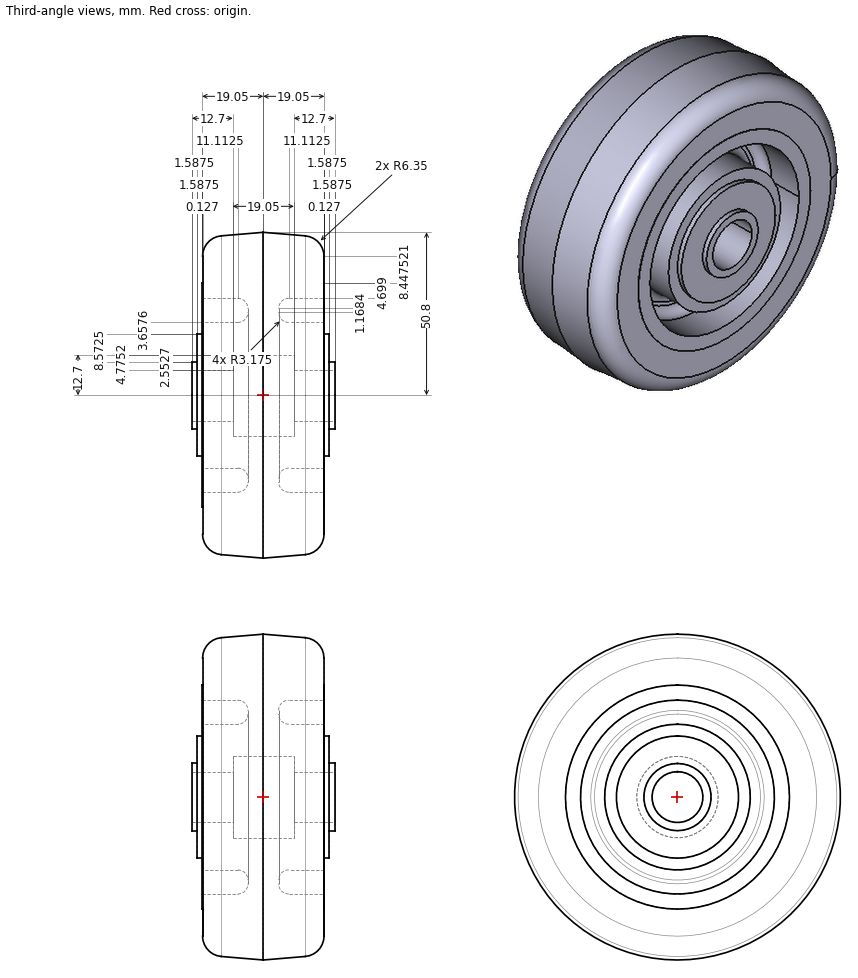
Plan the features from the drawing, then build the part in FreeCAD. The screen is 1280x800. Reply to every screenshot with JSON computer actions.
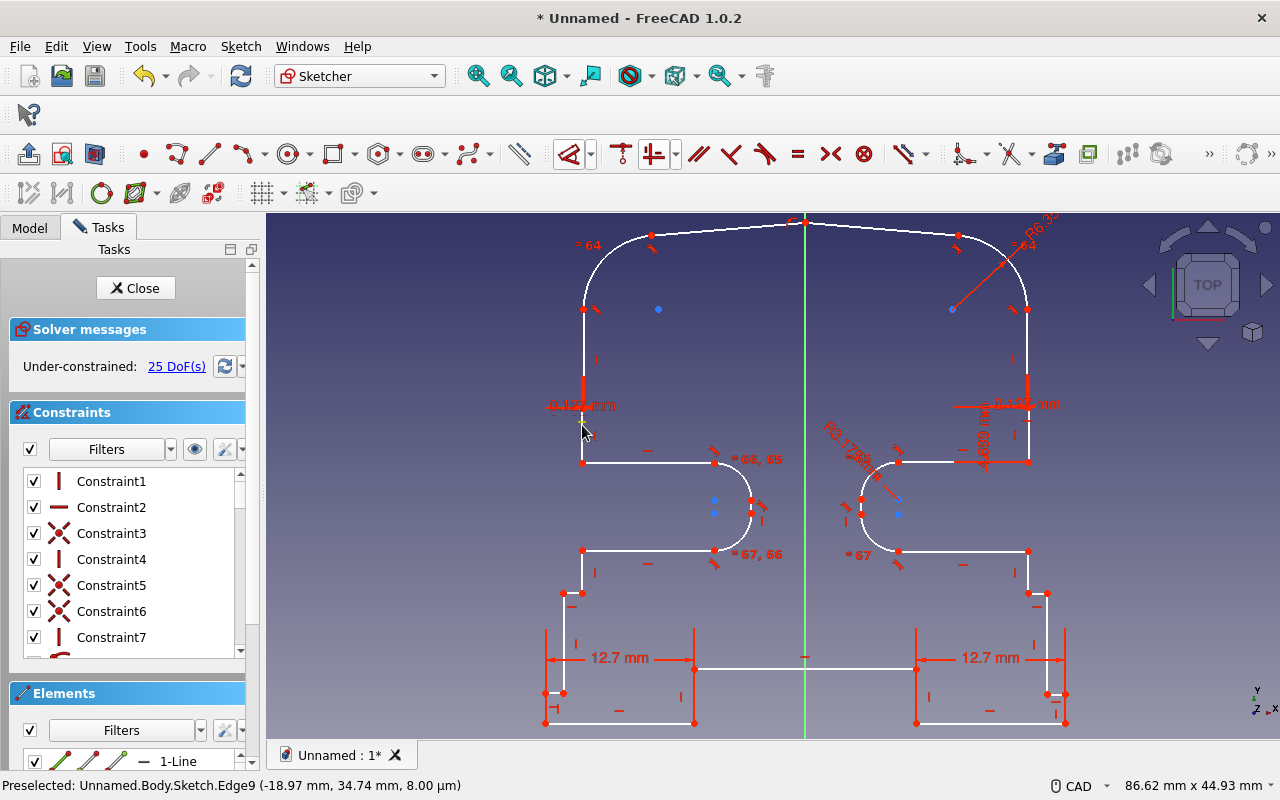
{"action": "left_click", "coordinate": [582, 447]}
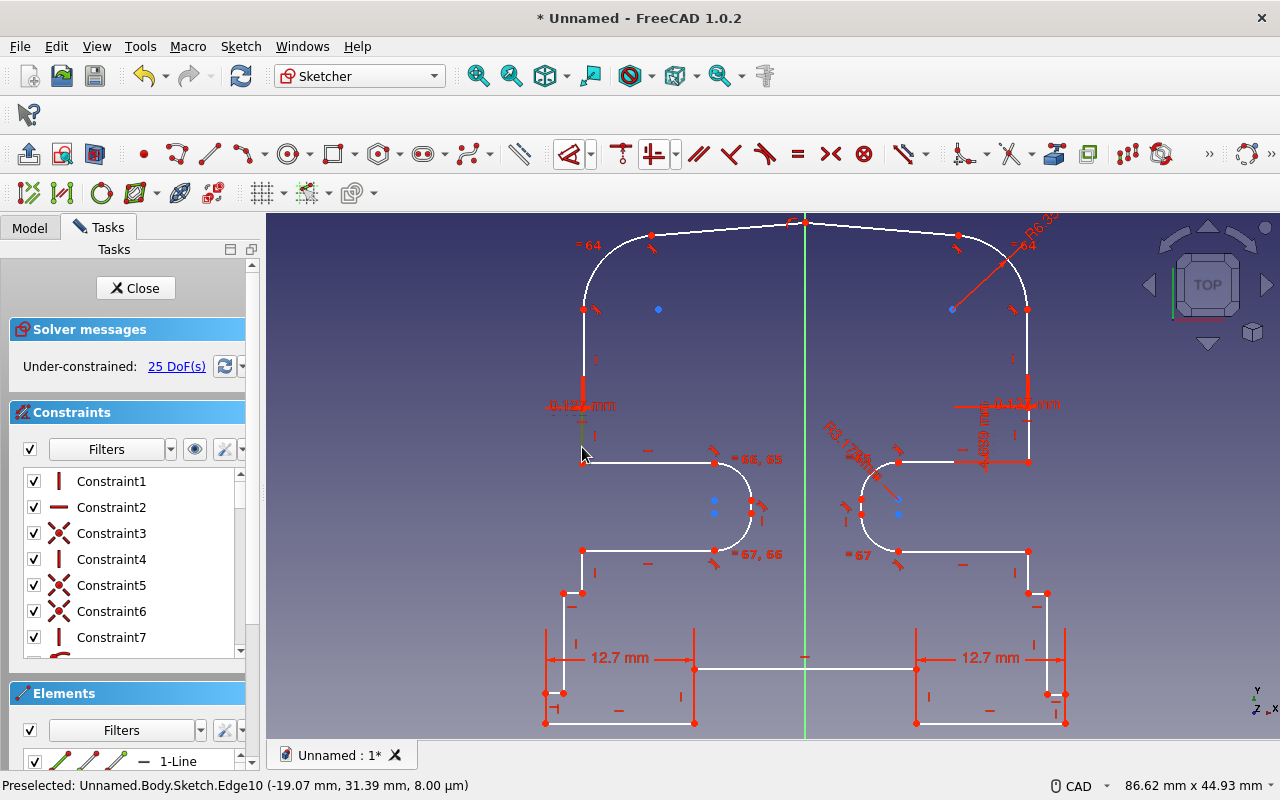
{"action": "left_click", "coordinate": [590, 154]}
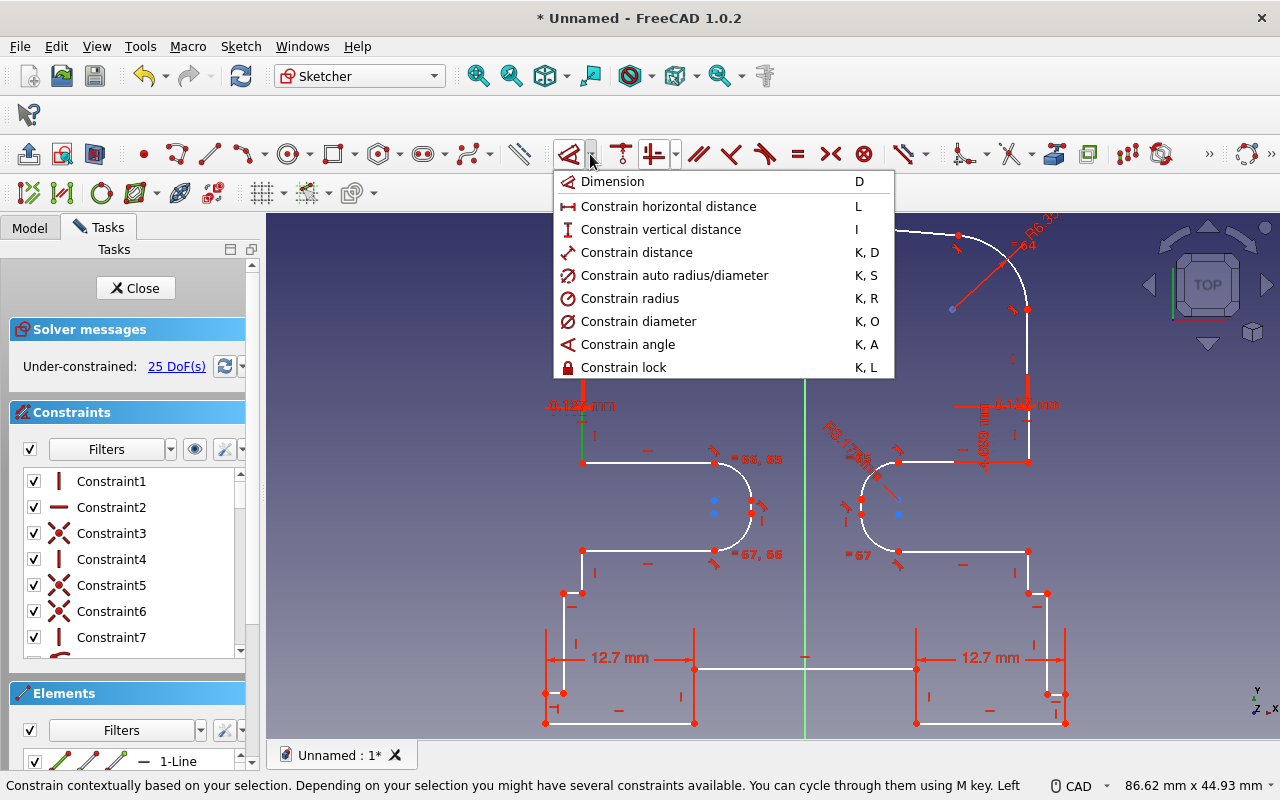
{"action": "left_click", "coordinate": [724, 230]}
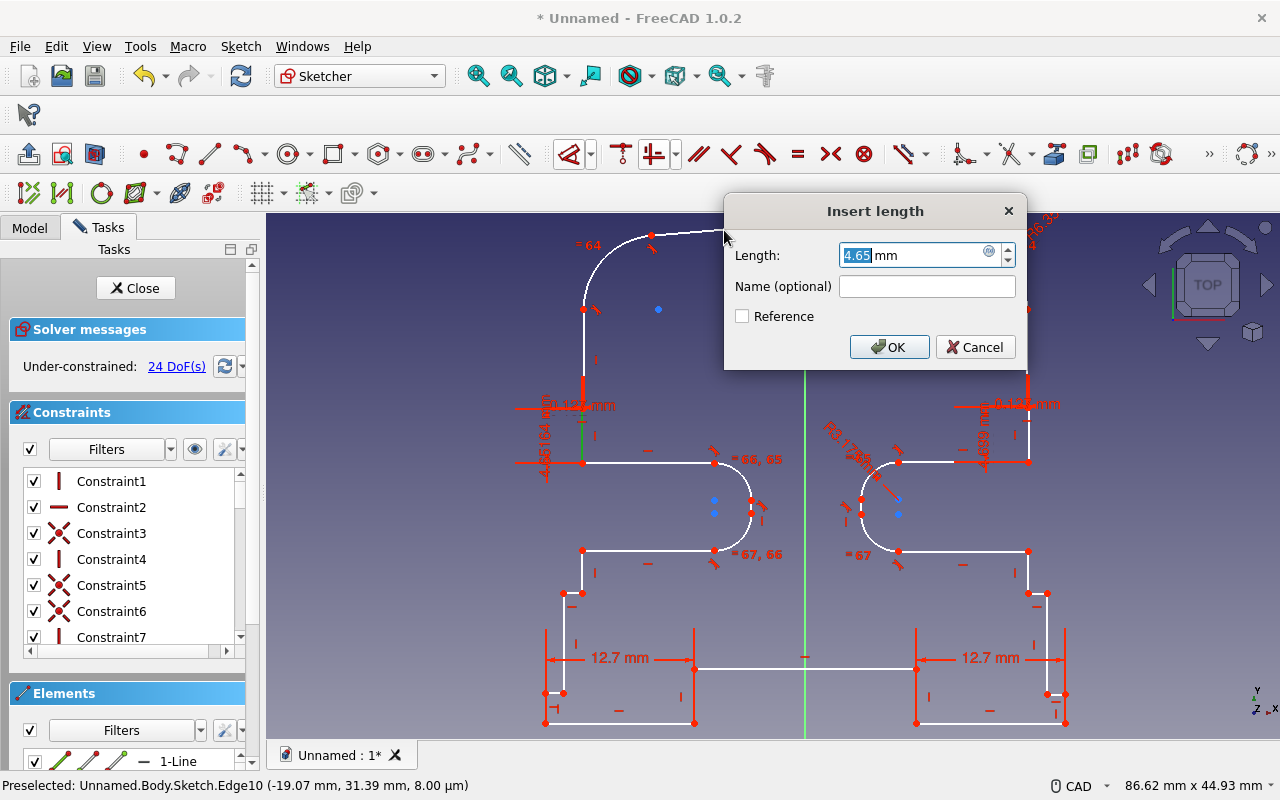
{"action": "type", "text": "4.699"}
{"action": "key", "text": "Return"}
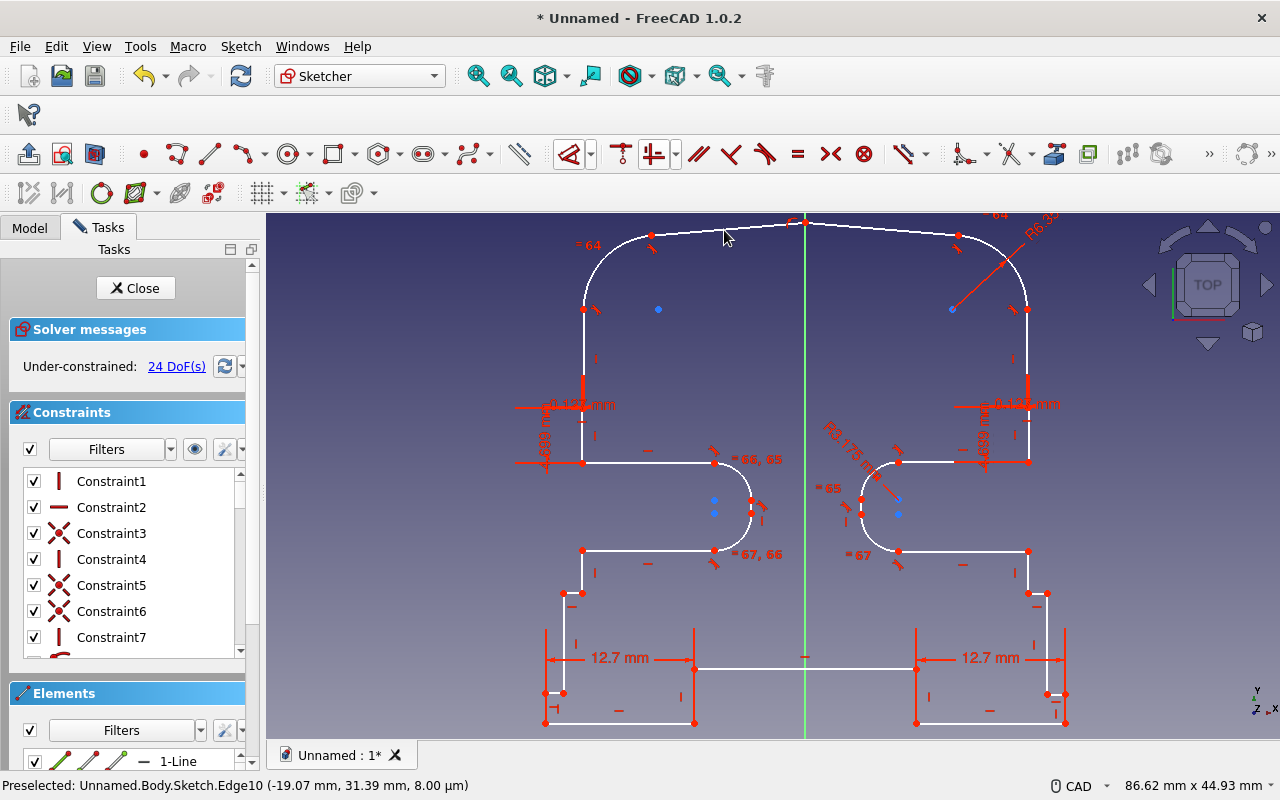
{"action": "left_click", "coordinate": [761, 669]}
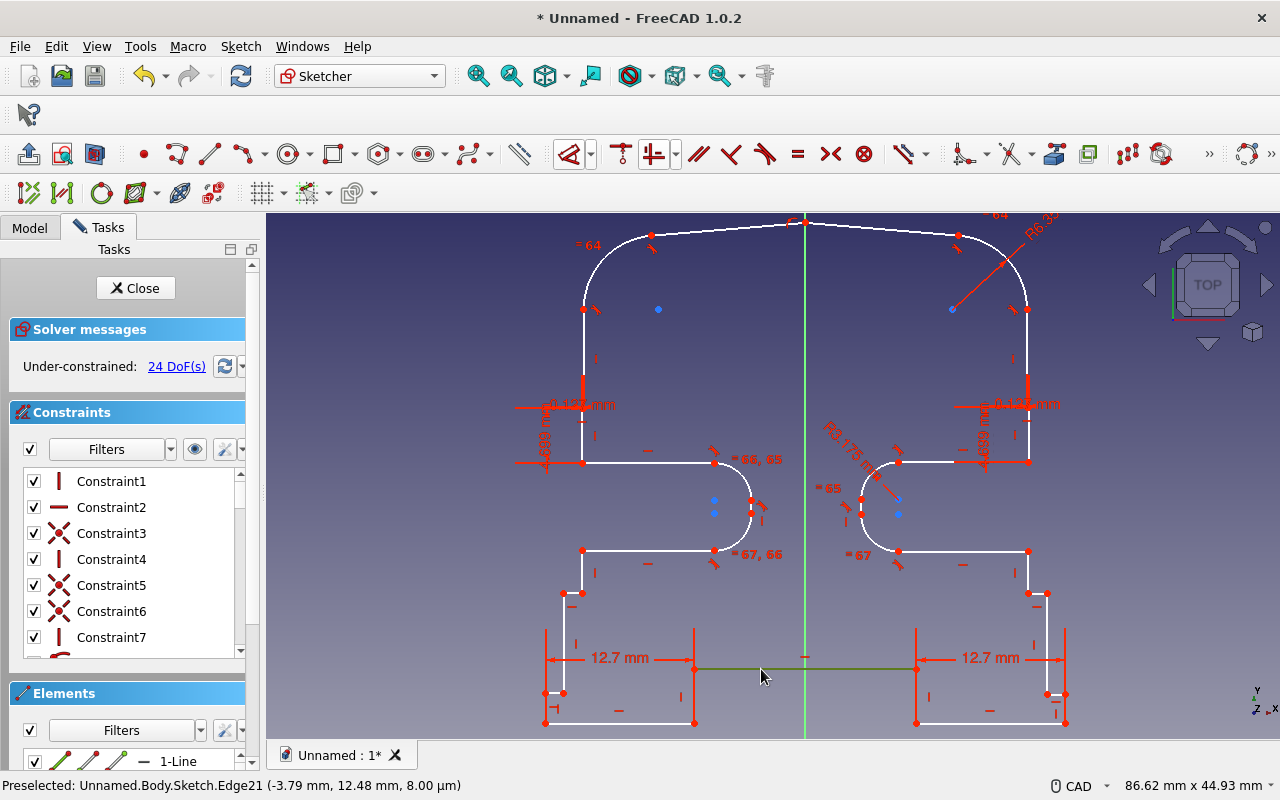
{"action": "left_click", "coordinate": [590, 154]}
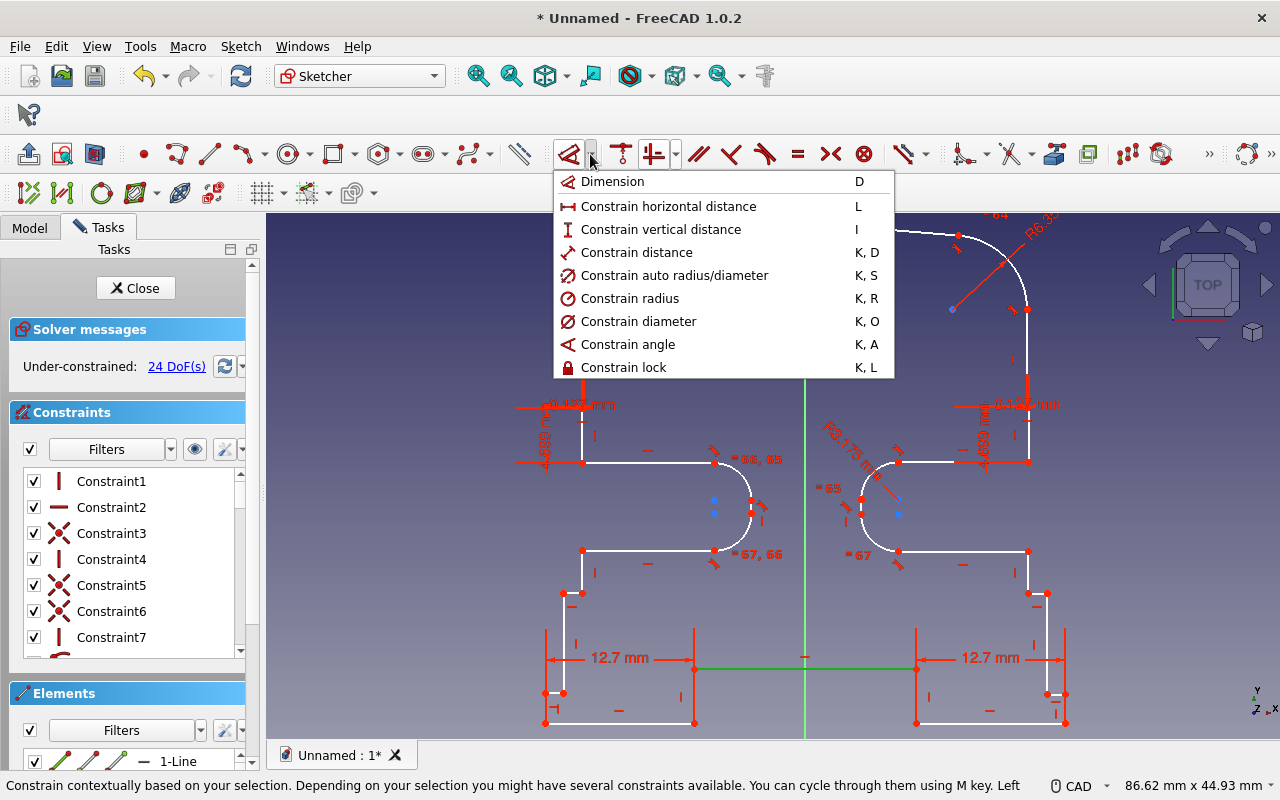
{"action": "left_click", "coordinate": [724, 206]}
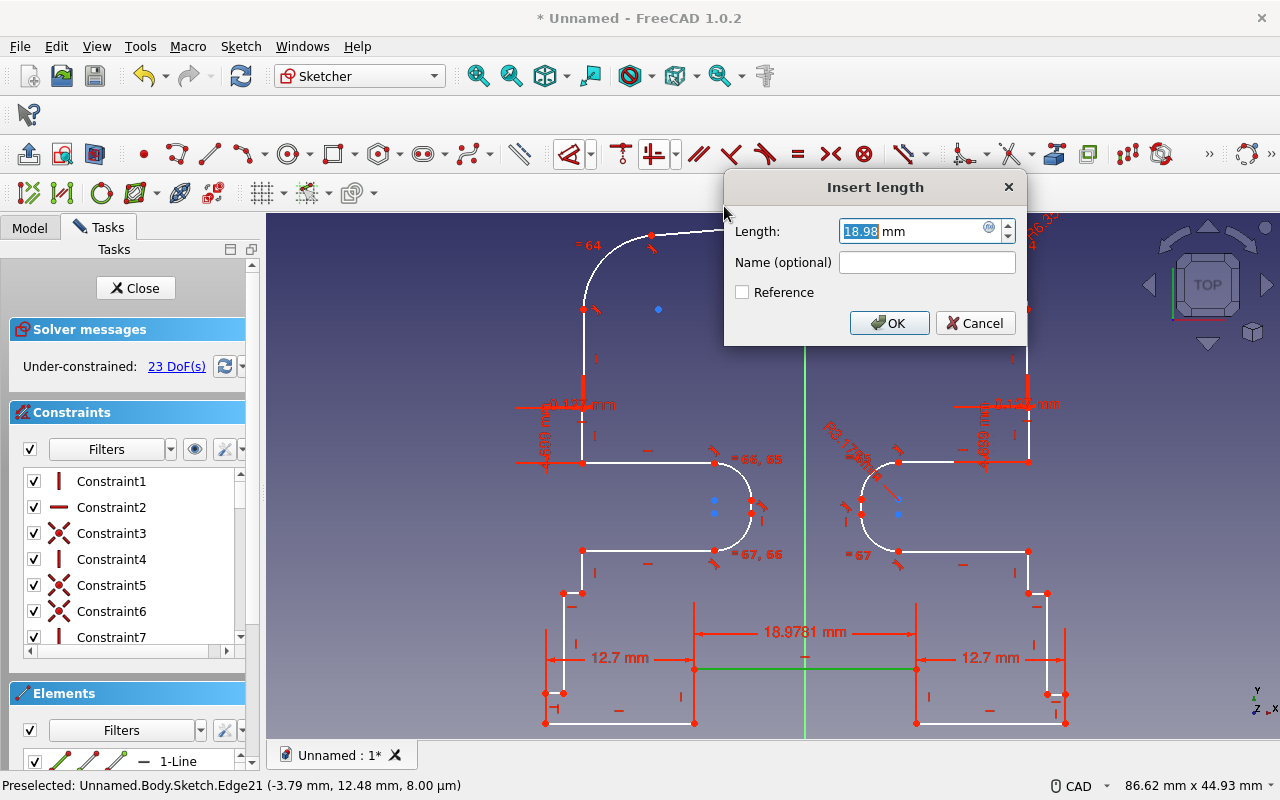
{"action": "type", "text": "19.05"}
{"action": "key", "text": "Return"}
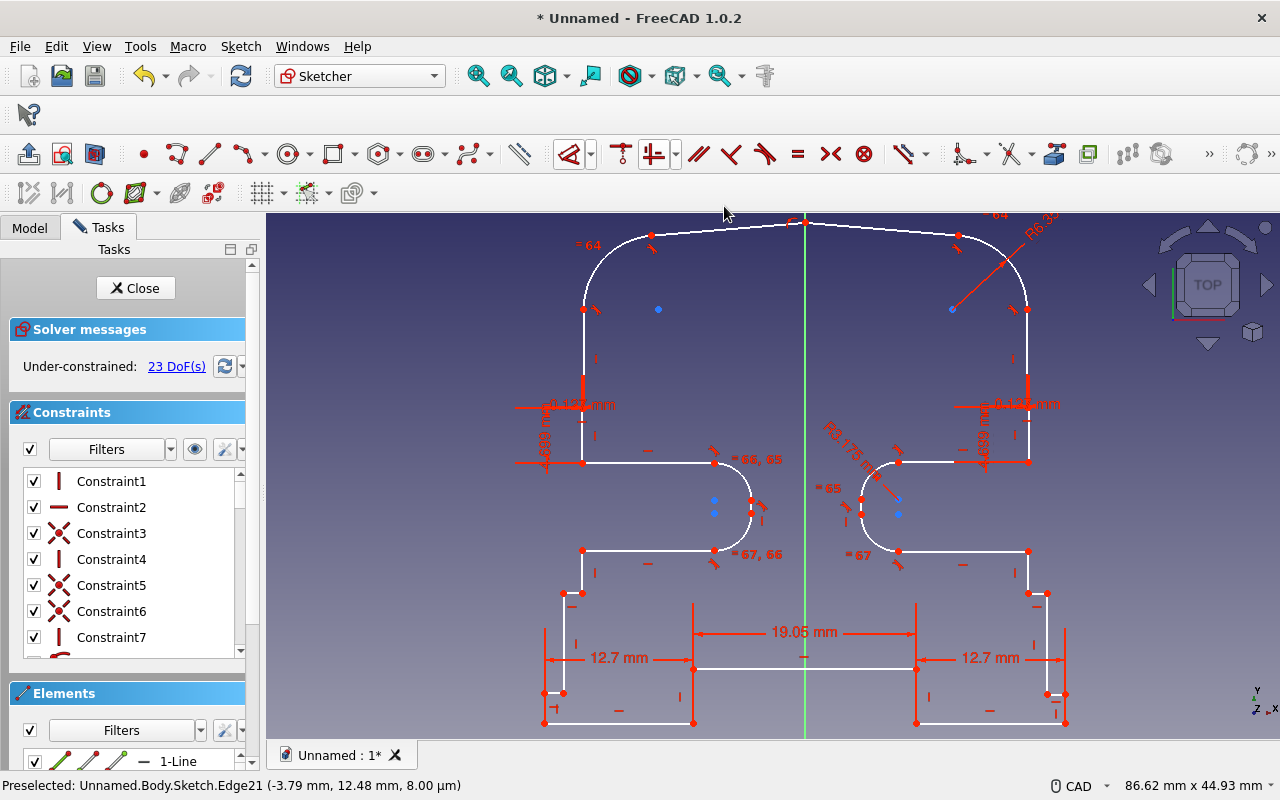
{"action": "scroll", "coordinate": [582, 425], "scroll_direction": "down", "scroll_amount": 3}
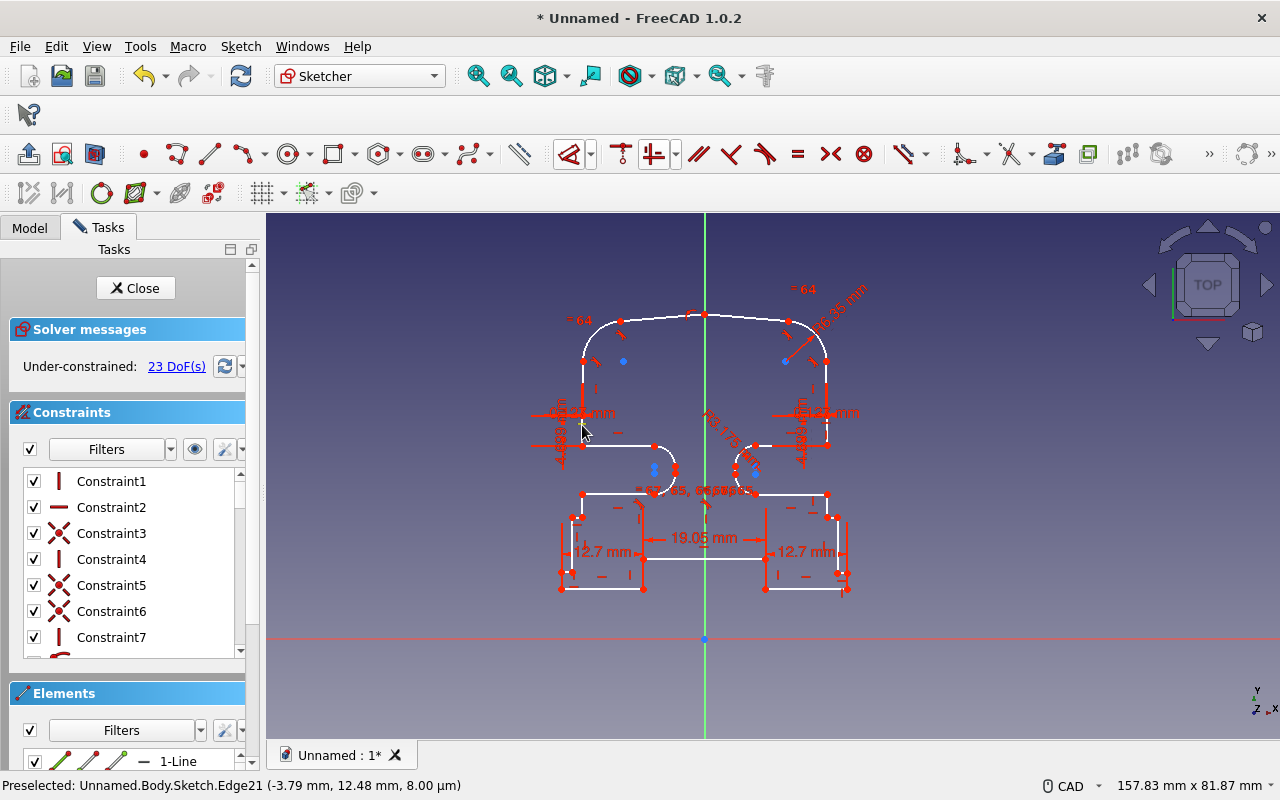
{"action": "left_click", "coordinate": [705, 314]}